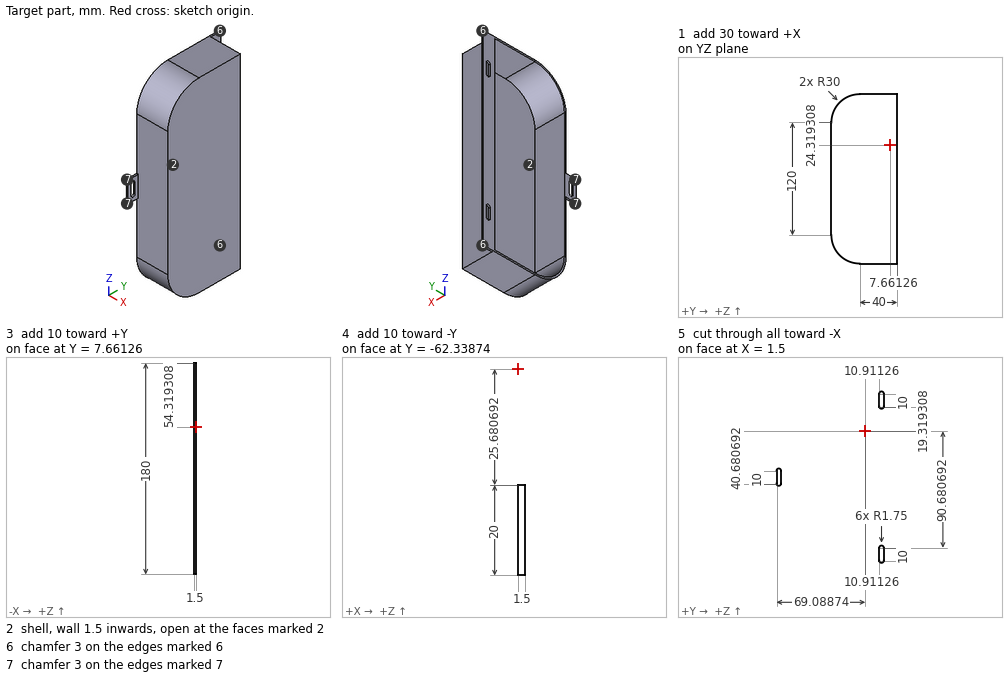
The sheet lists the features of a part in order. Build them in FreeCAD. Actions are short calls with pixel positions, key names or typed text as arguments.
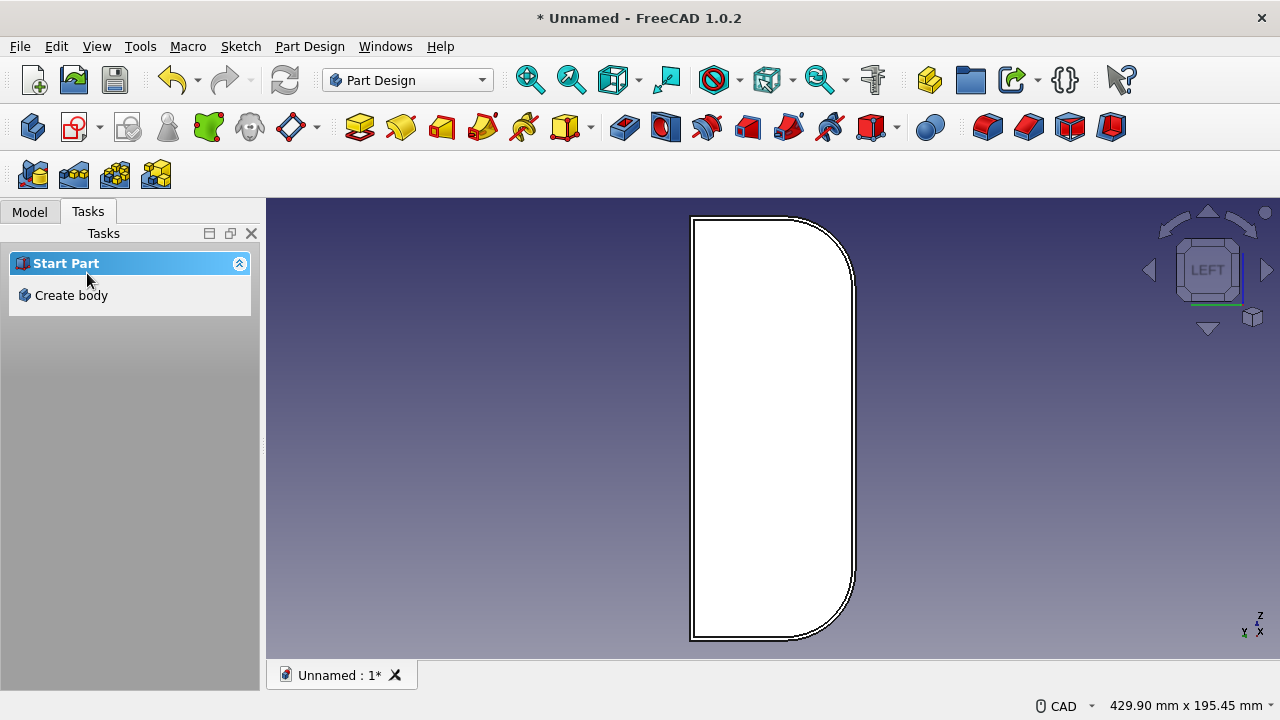
key(4)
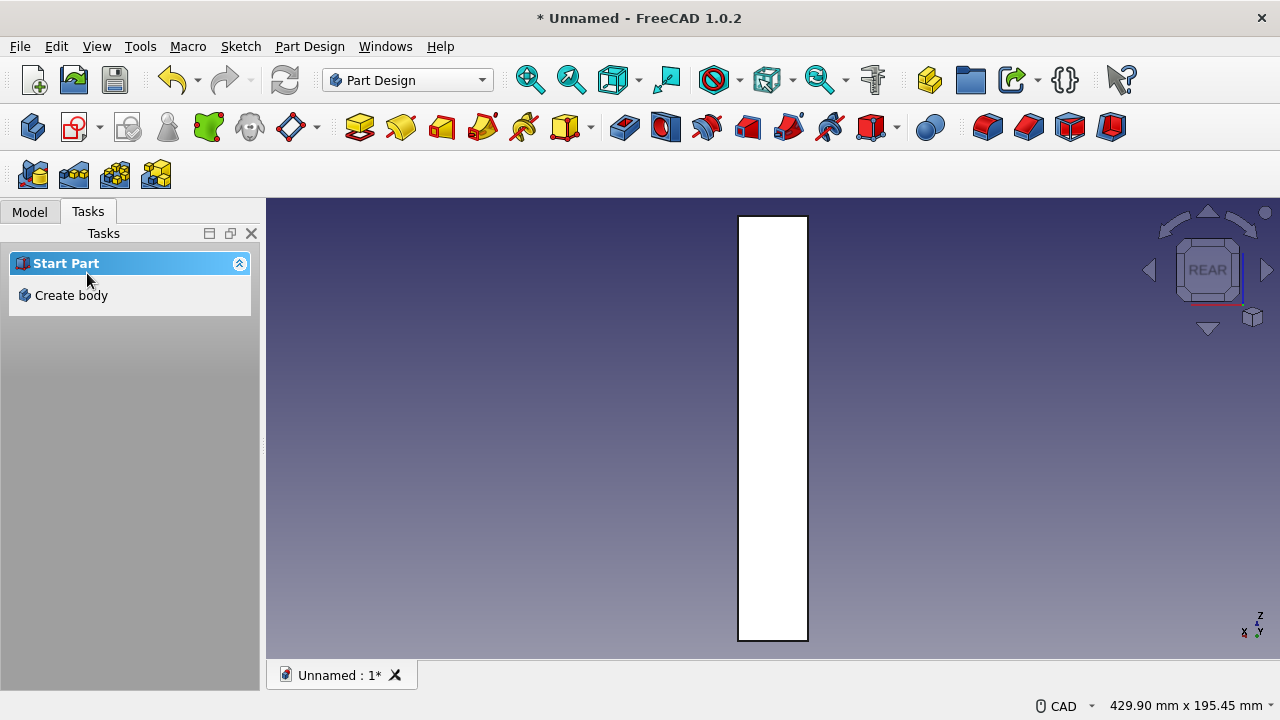
click(773, 549)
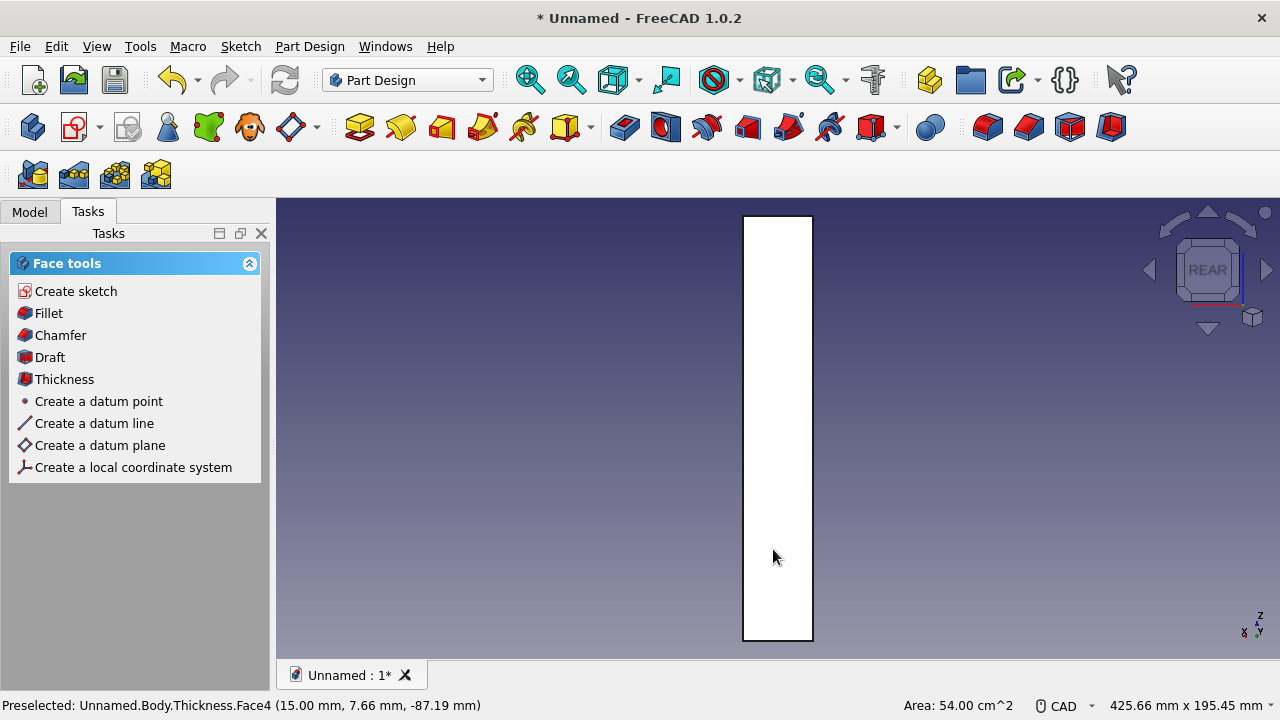
click(74, 128)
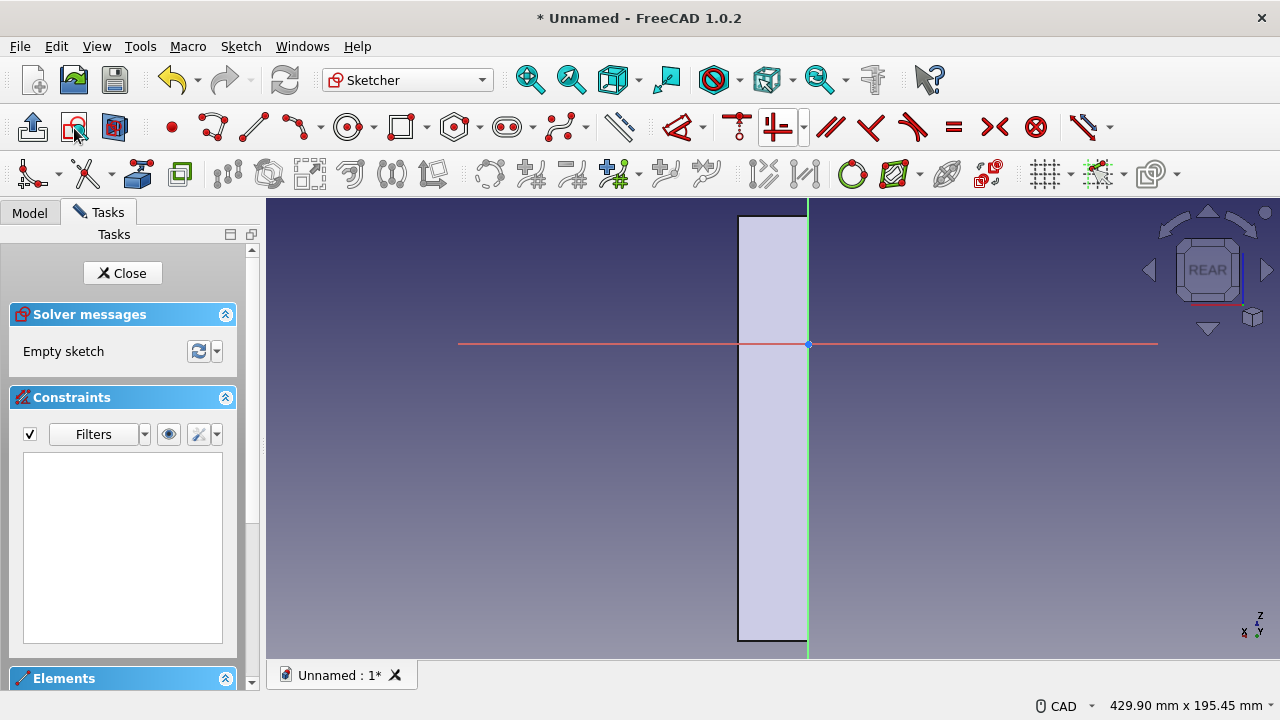
scroll(497, 429, down, 2)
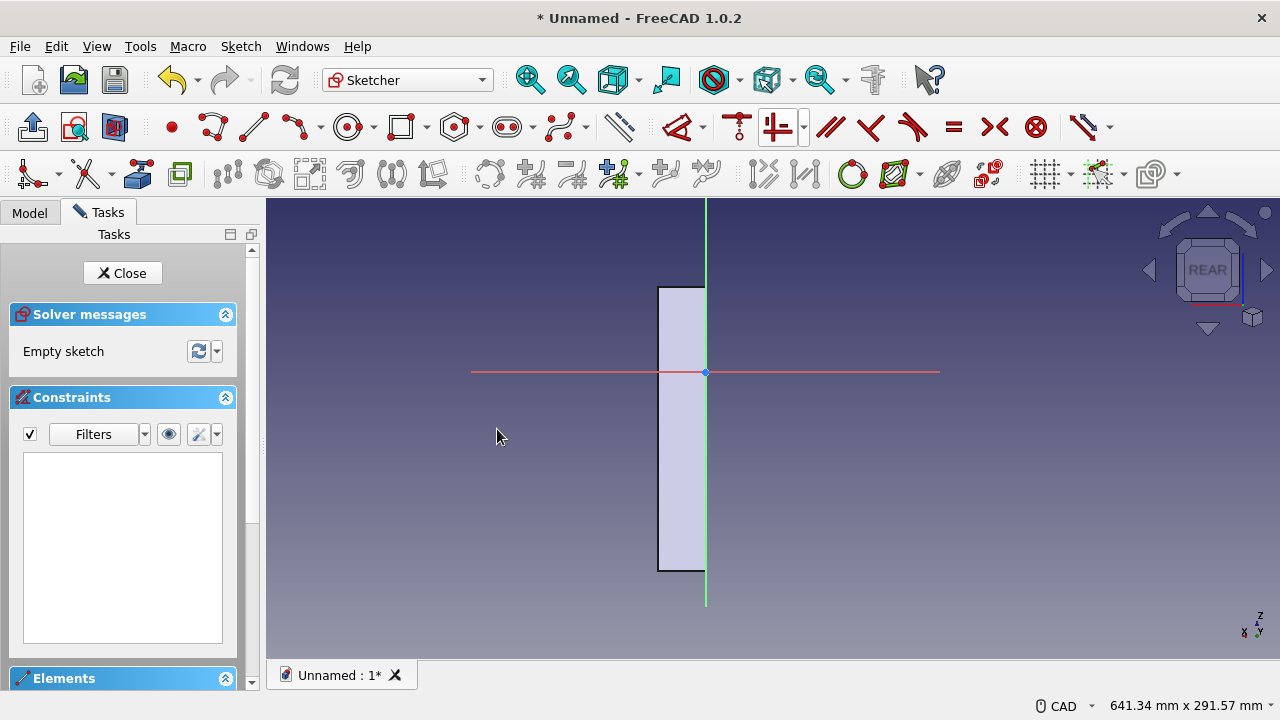
click(400, 128)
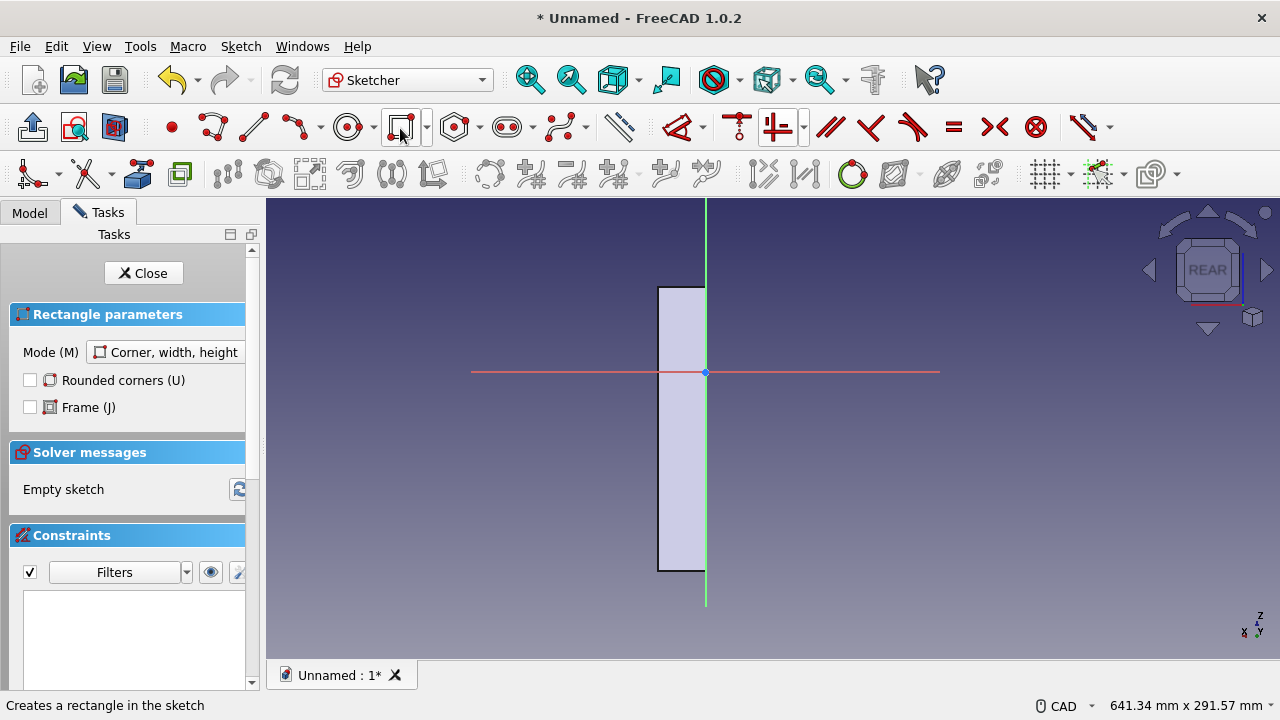
scroll(703, 287, up, 10)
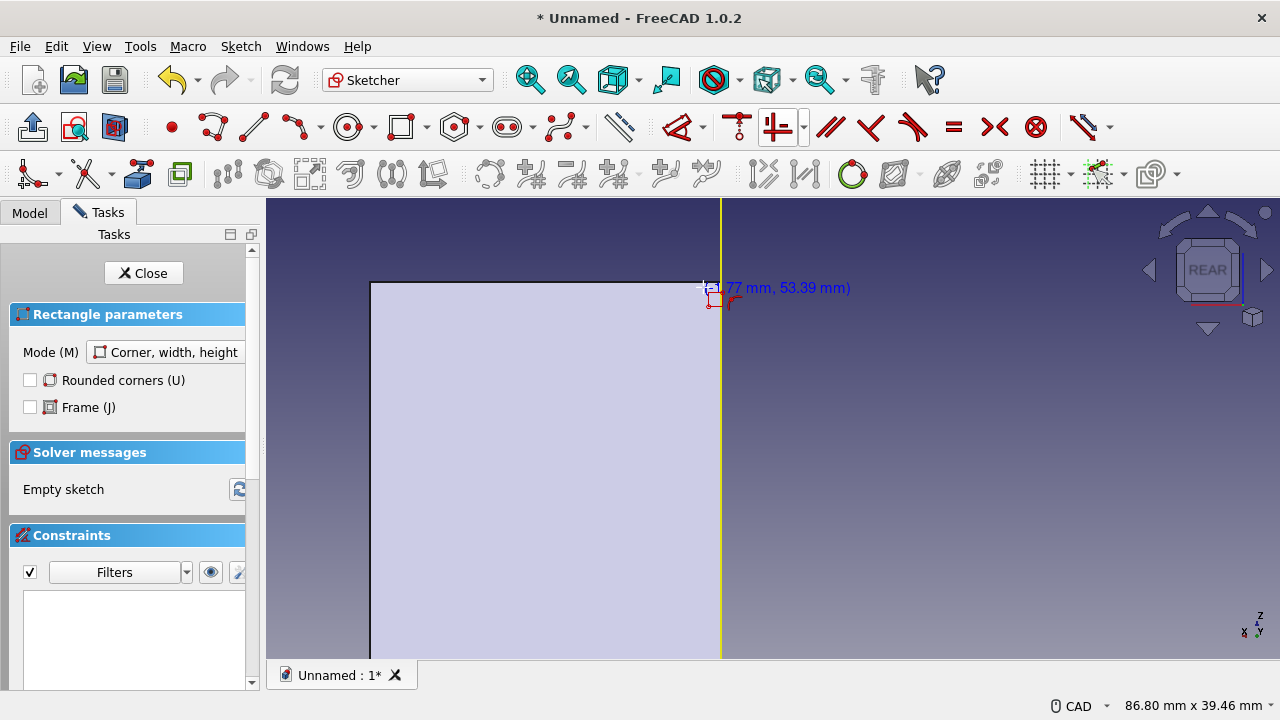
click(703, 282)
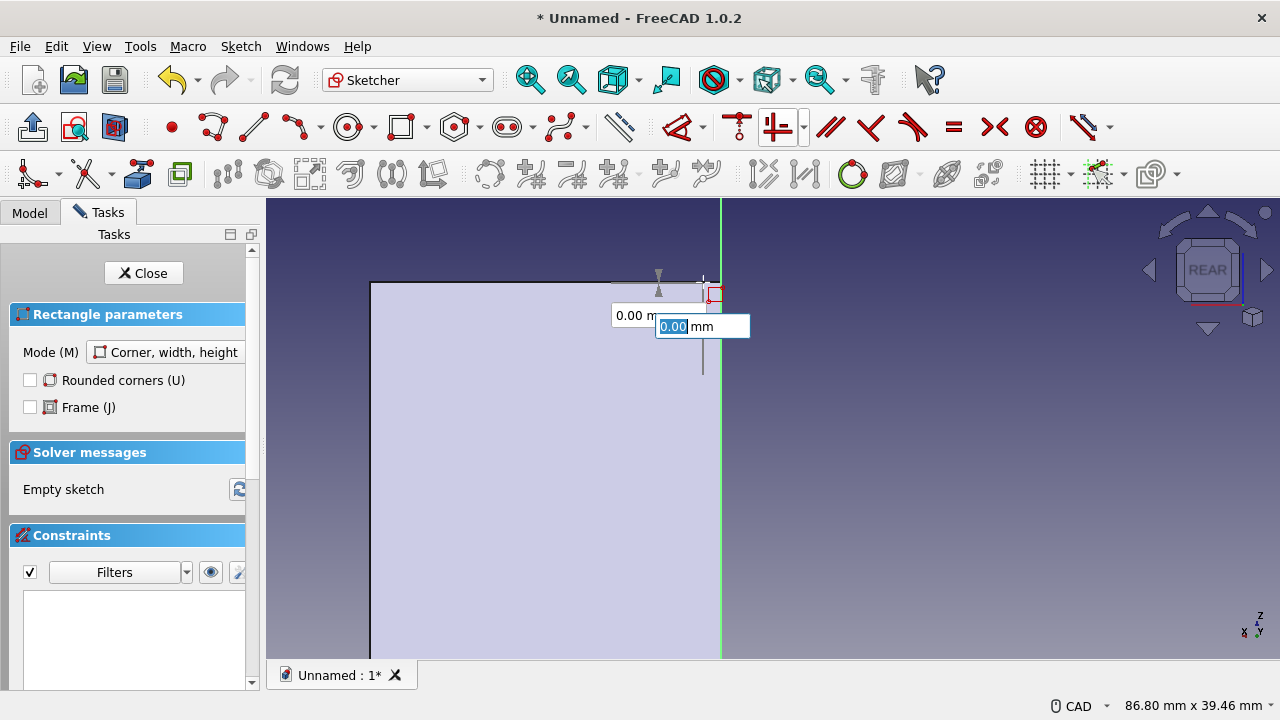
scroll(703, 287, down, 10)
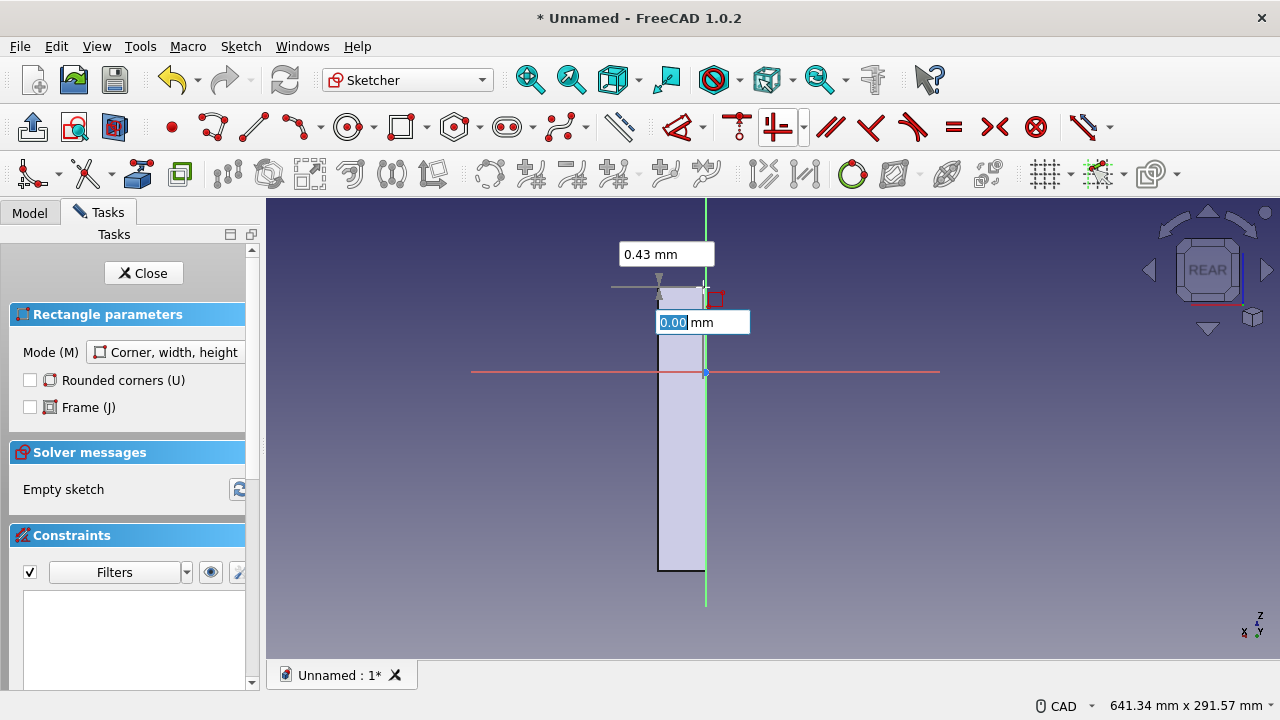
click(706, 571)
key(Escape)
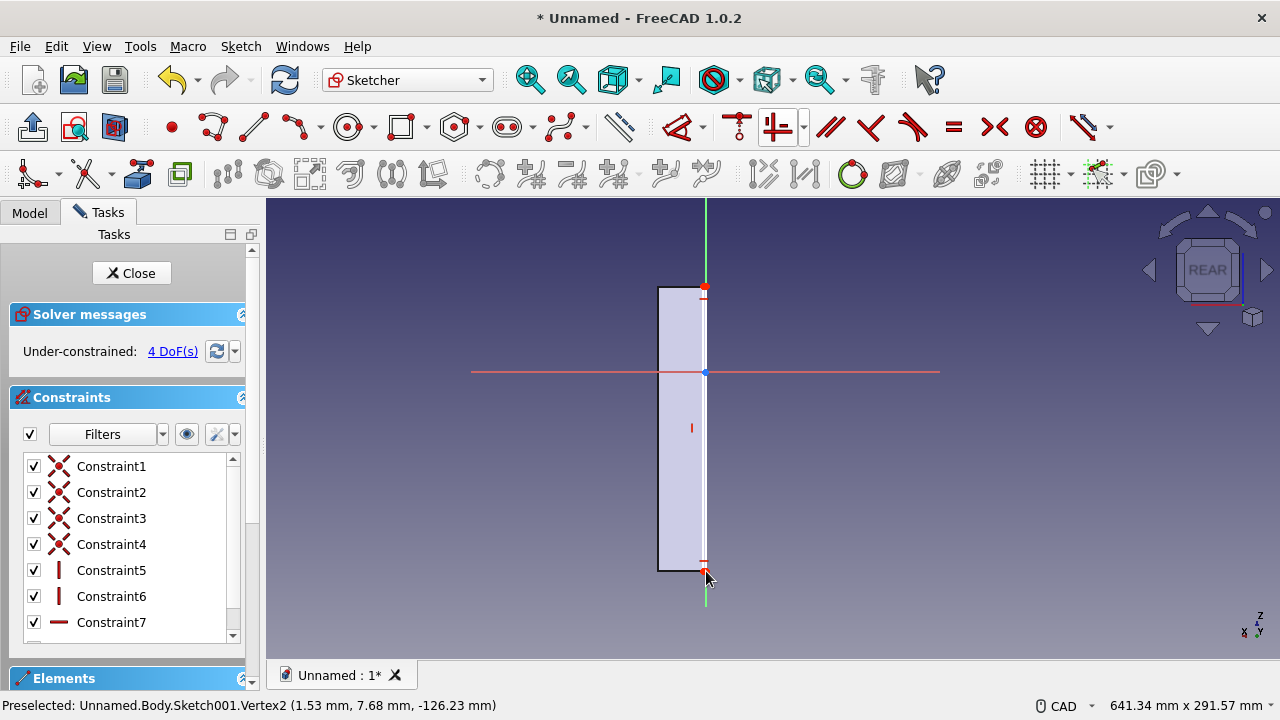
scroll(706, 572, up, 8)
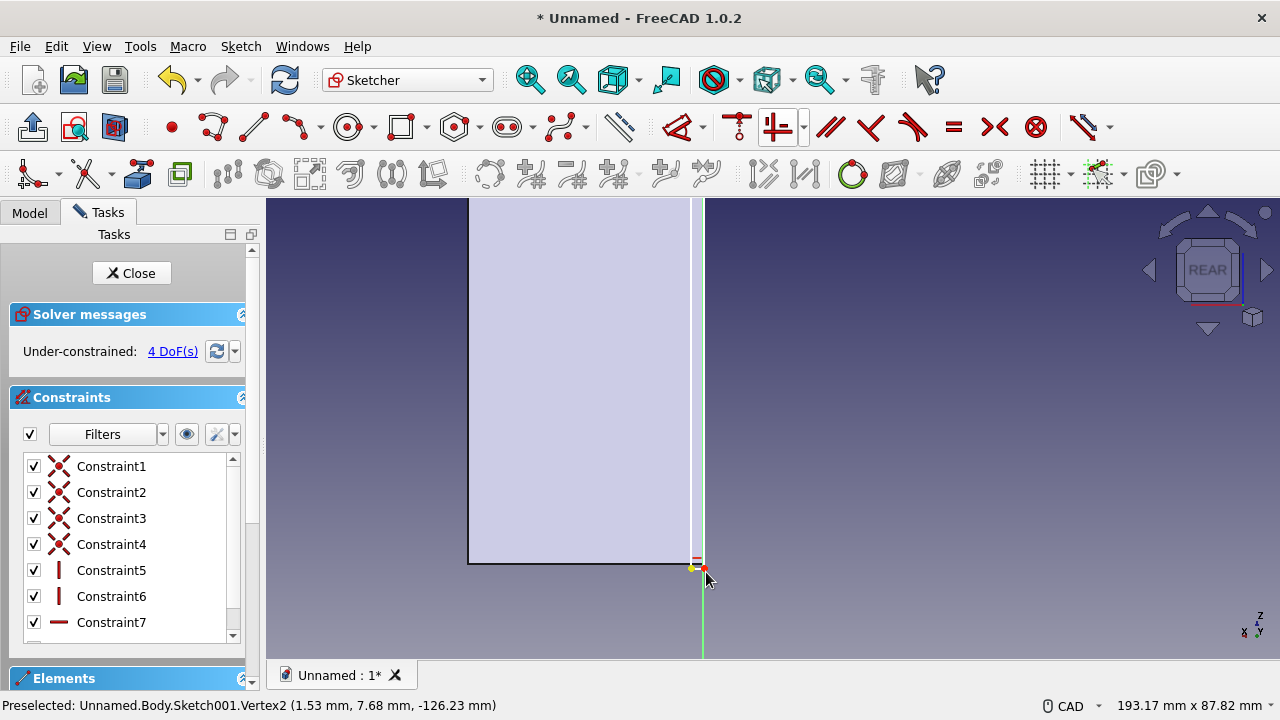
click(704, 569)